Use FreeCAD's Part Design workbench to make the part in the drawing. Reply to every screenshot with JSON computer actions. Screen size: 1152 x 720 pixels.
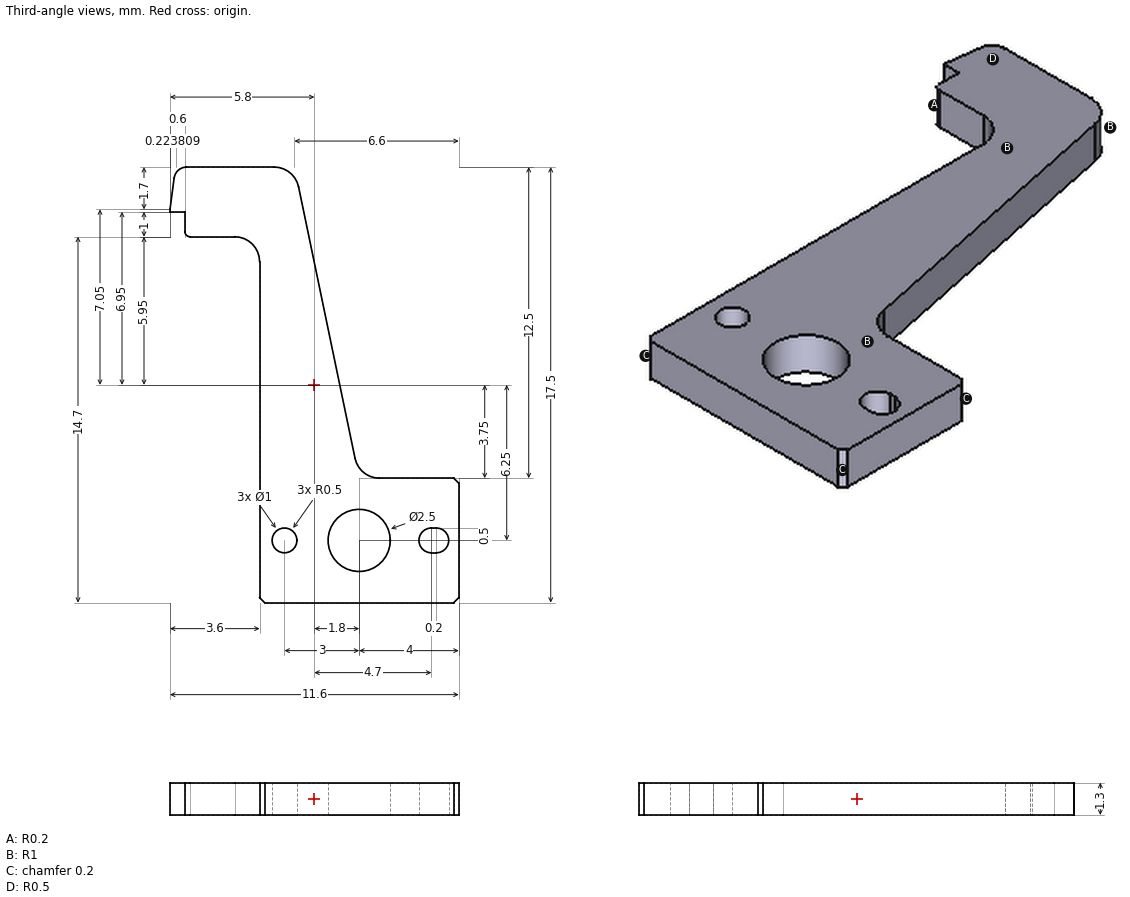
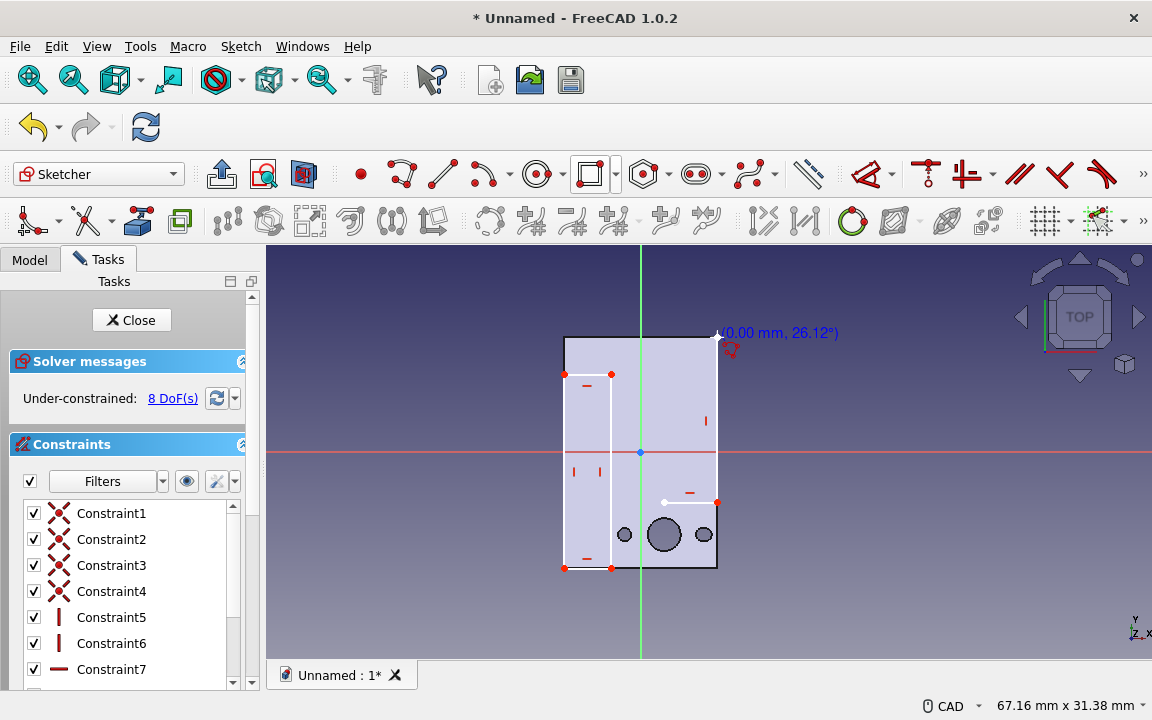
{"action": "scroll", "coordinate": [630, 337], "scroll_direction": "up", "scroll_amount": 3}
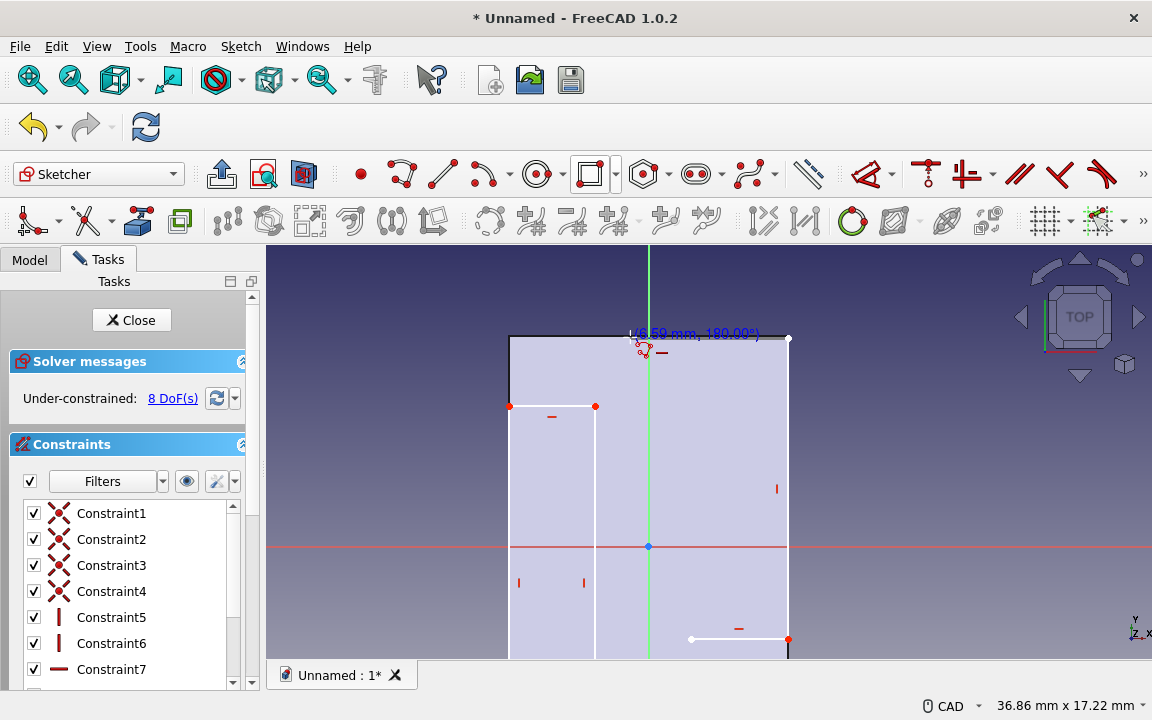
{"action": "left_click", "coordinate": [630, 337]}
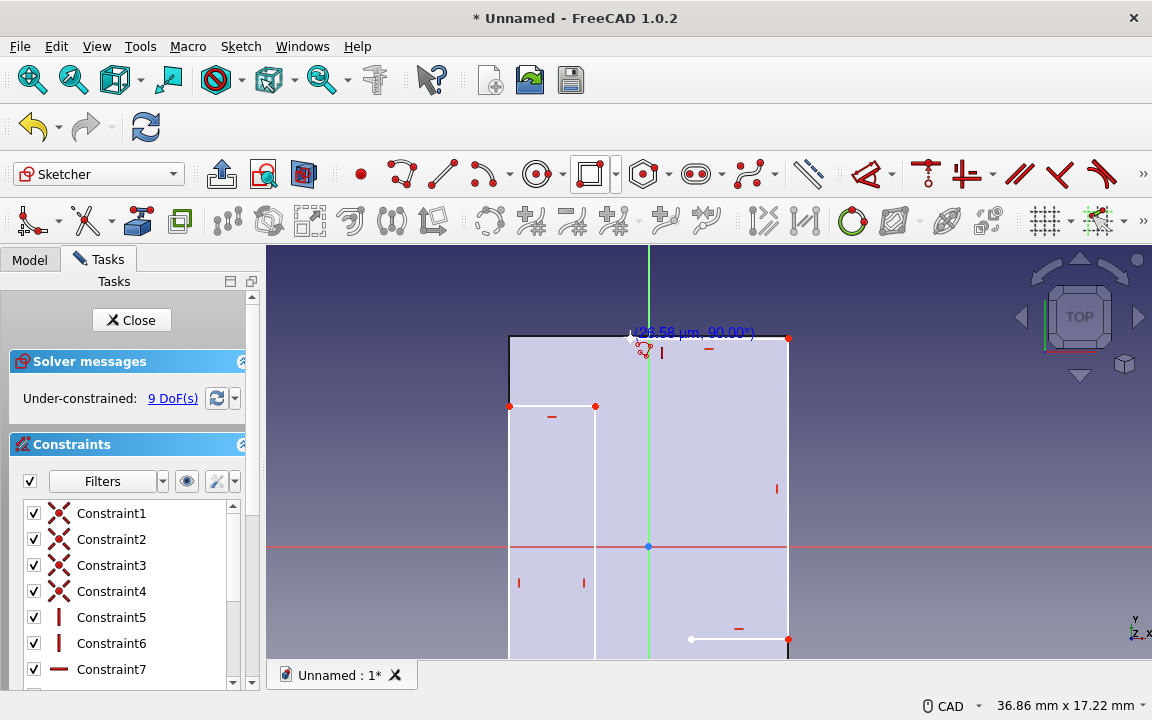
{"action": "scroll", "coordinate": [630, 337], "scroll_direction": "down", "scroll_amount": 3}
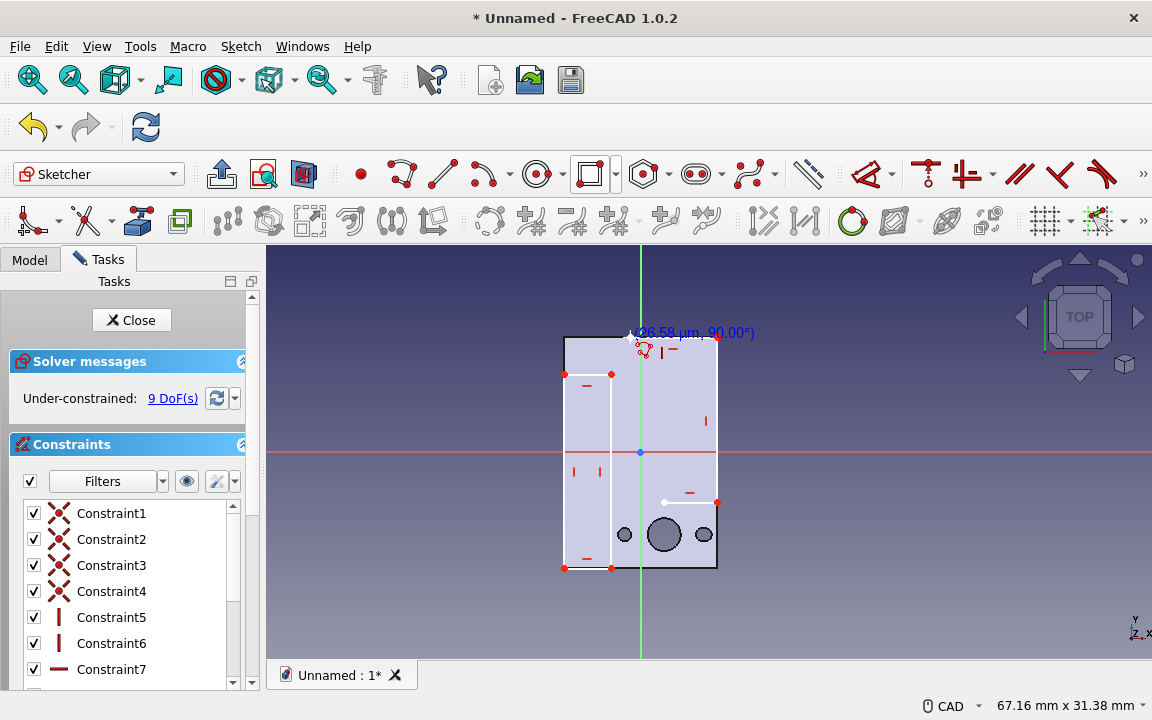
{"action": "left_click", "coordinate": [664, 503]}
{"action": "key", "text": "Escape"}
{"action": "key", "text": "Escape"}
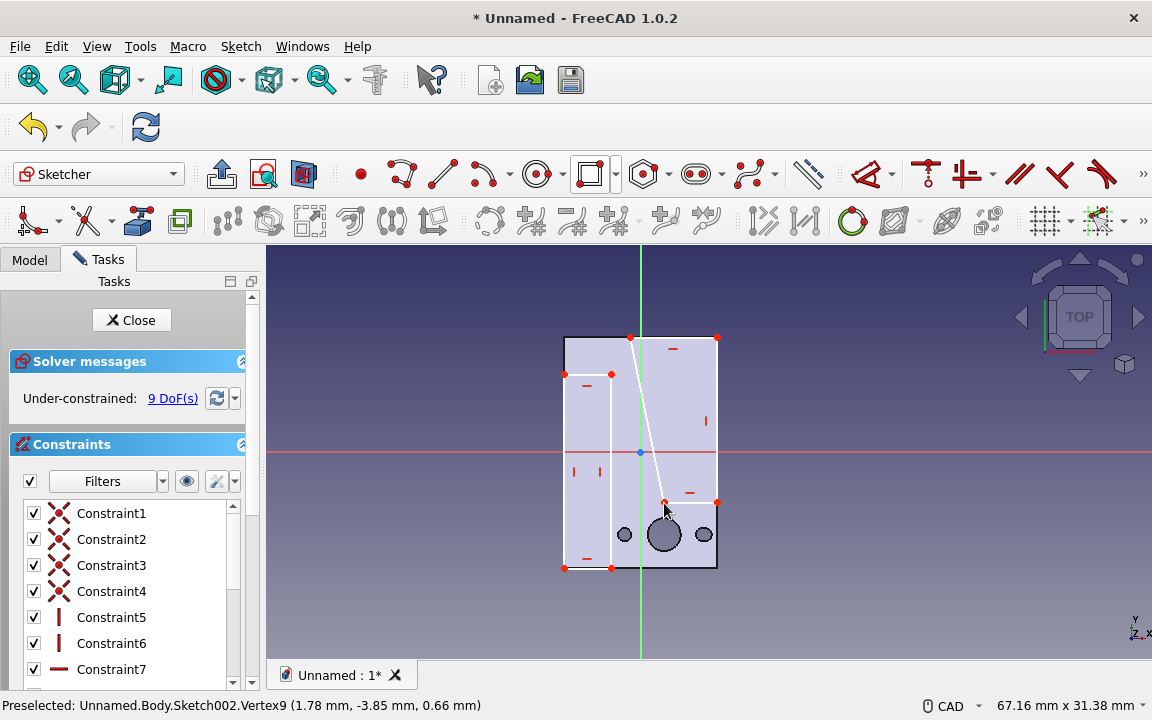
{"action": "key", "text": "d"}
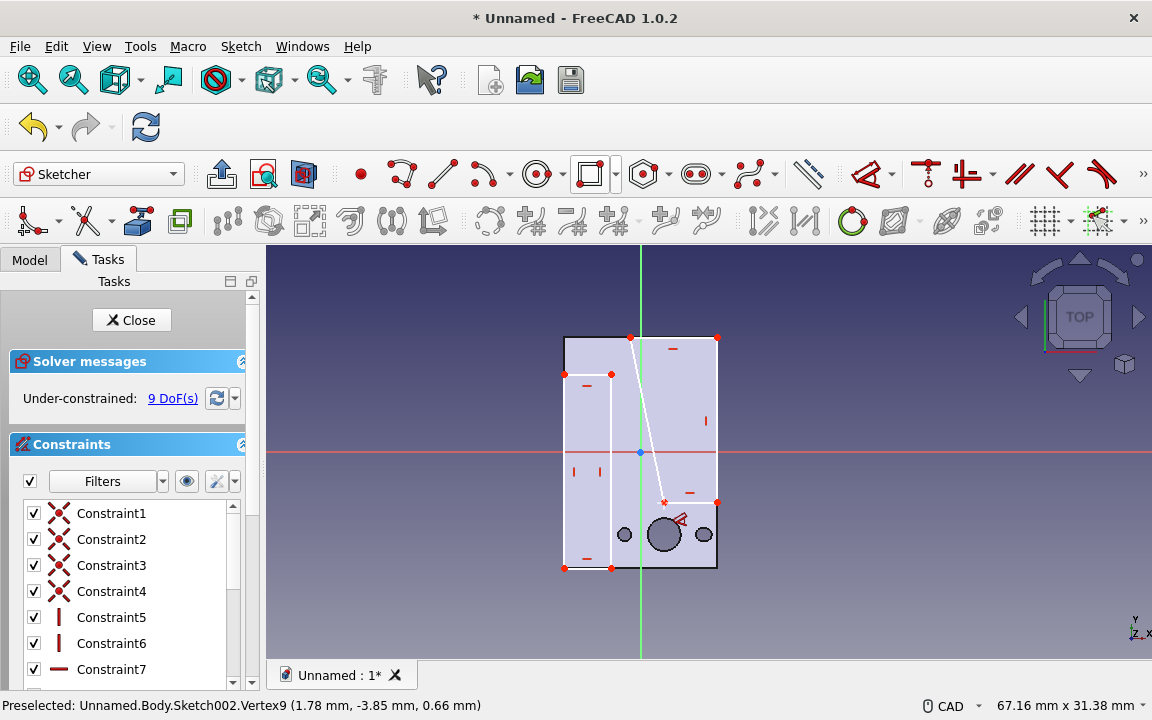
{"action": "left_click", "coordinate": [680, 503]}
{"action": "left_click", "coordinate": [690, 537]}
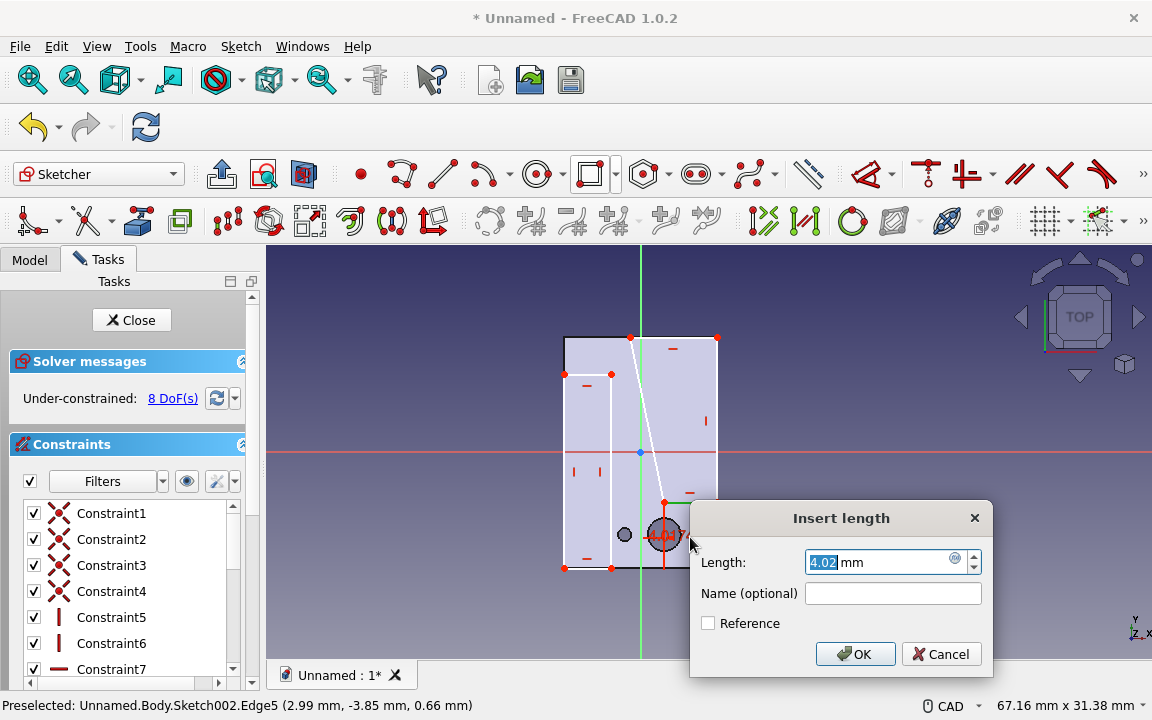
{"action": "type", "text": "4"}
{"action": "key", "text": "Return"}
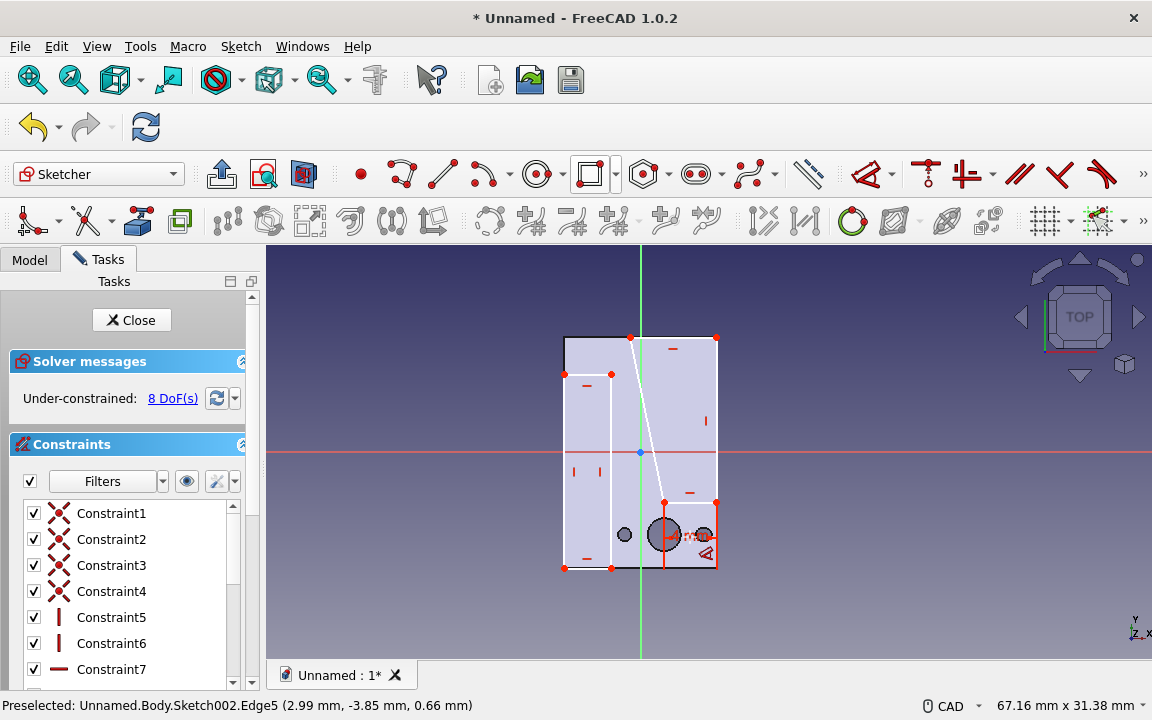
{"action": "left_click", "coordinate": [578, 569]}
{"action": "left_click", "coordinate": [588, 603]}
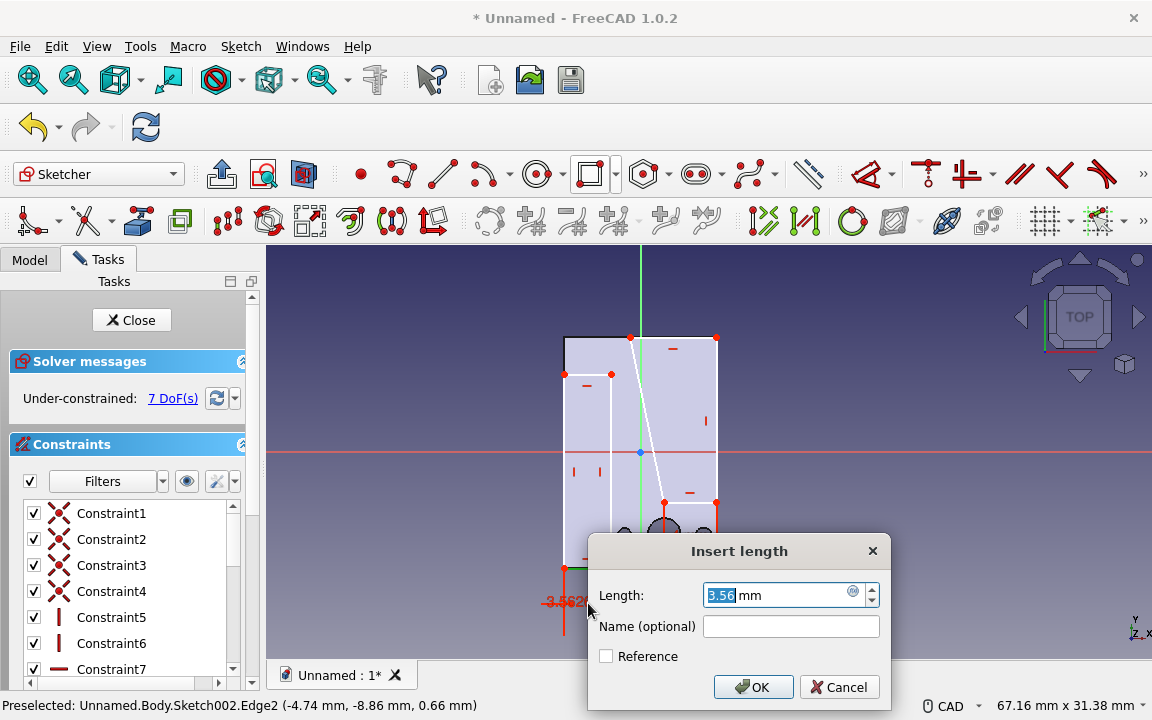
{"action": "type", "text": "3.6"}
{"action": "key", "text": "Return"}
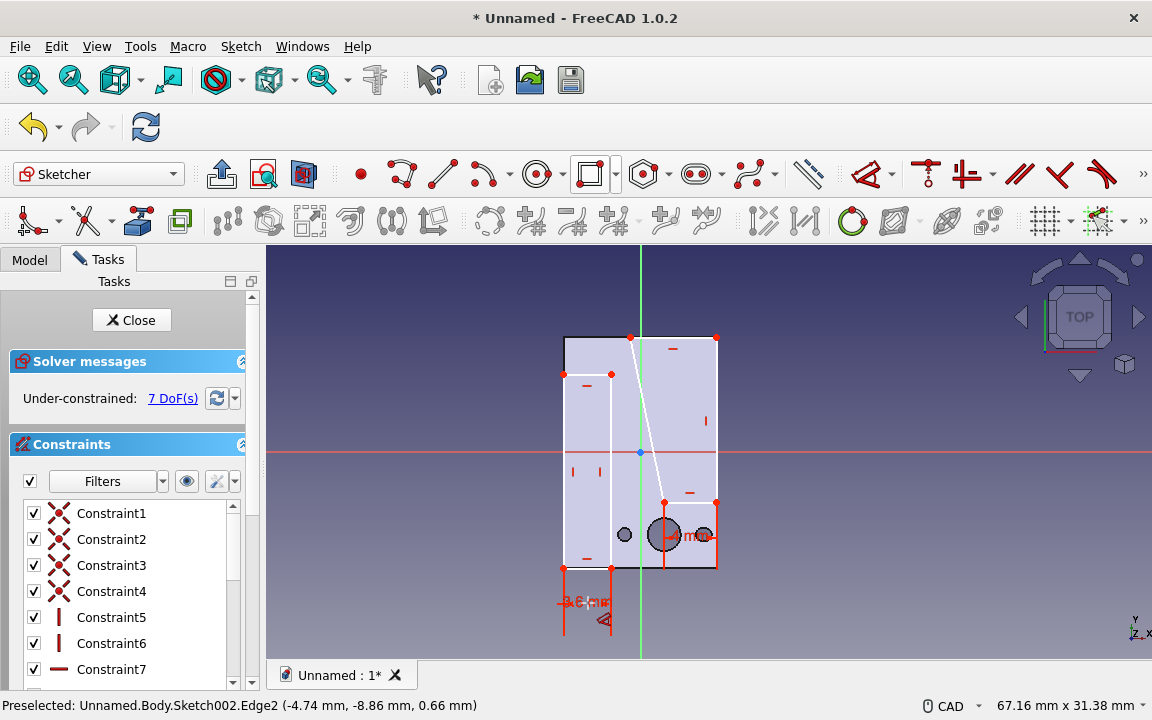
{"action": "left_click", "coordinate": [691, 338]}
{"action": "left_click", "coordinate": [673, 304]}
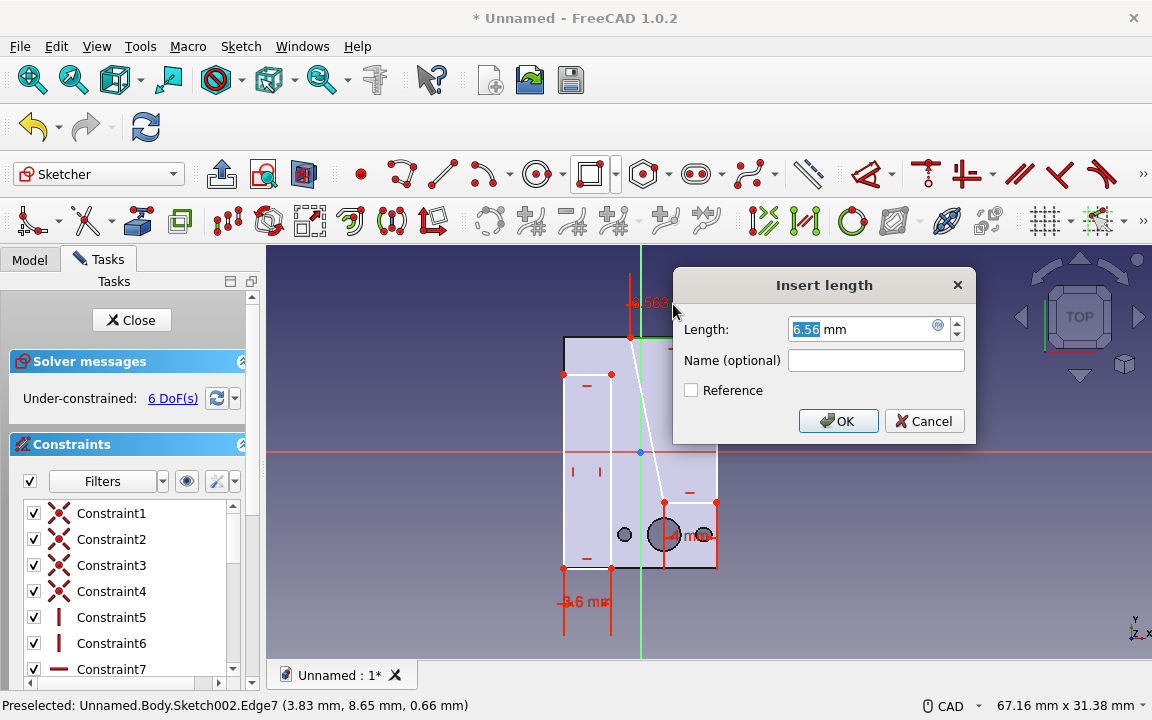
{"action": "type", "text": "6.6"}
{"action": "key", "text": "Return"}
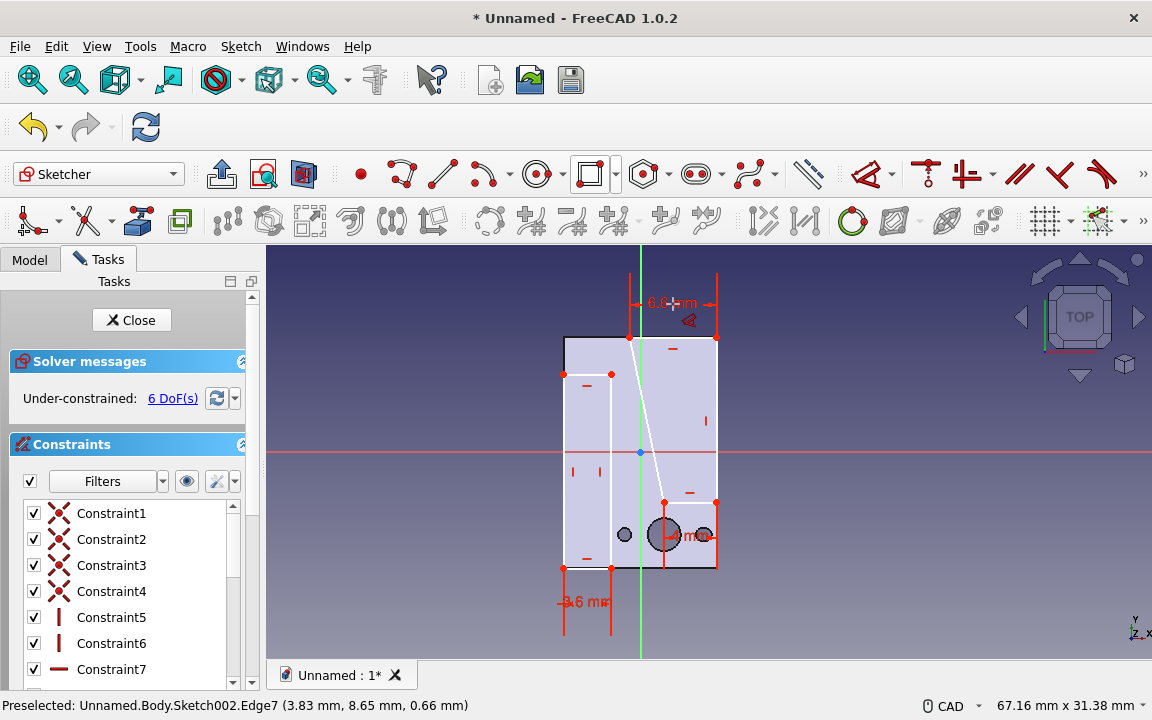
{"action": "left_click", "coordinate": [564, 433]}
{"action": "left_click", "coordinate": [530, 472]}